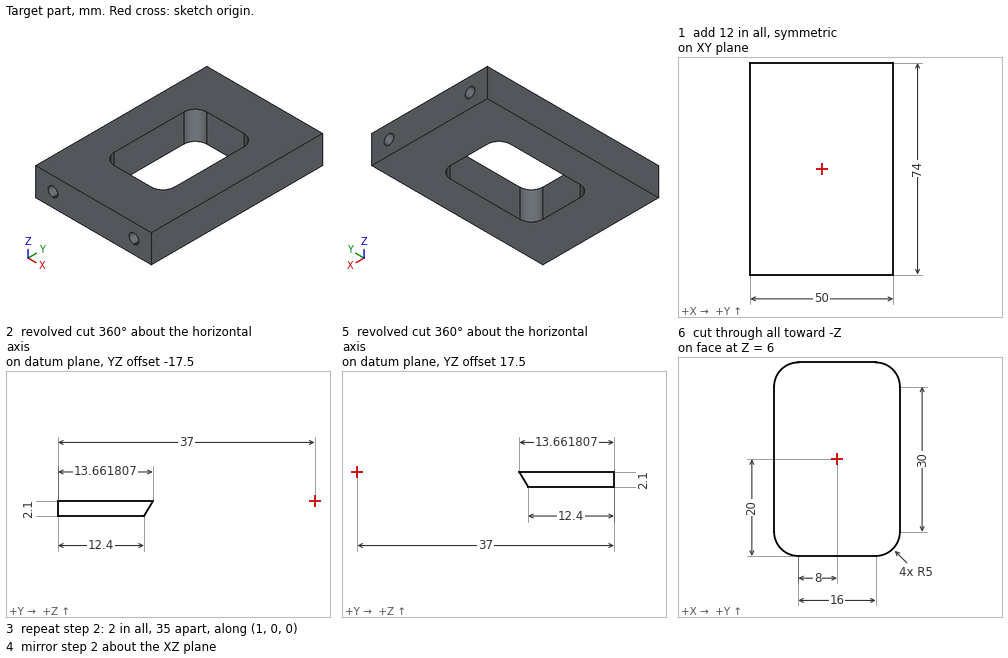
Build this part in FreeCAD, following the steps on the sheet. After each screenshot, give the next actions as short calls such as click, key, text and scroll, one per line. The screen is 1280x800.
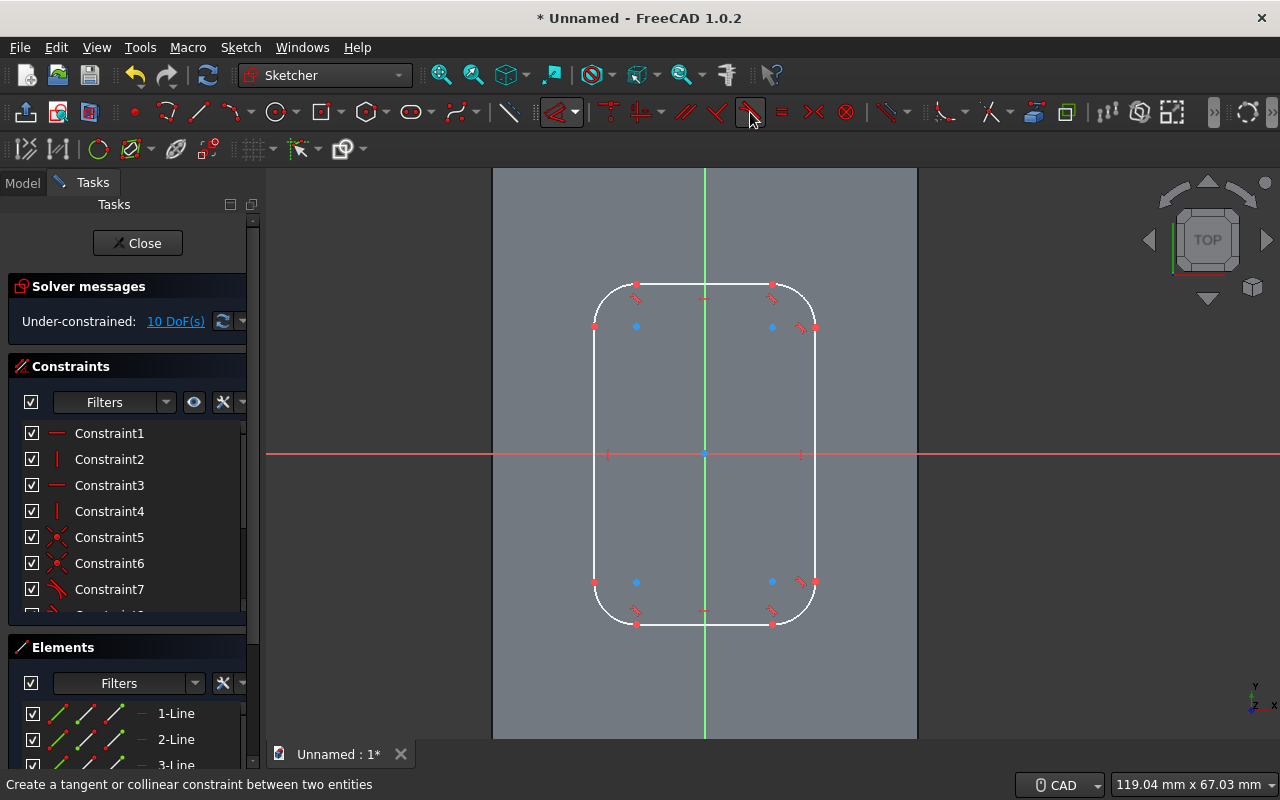
click(594, 403)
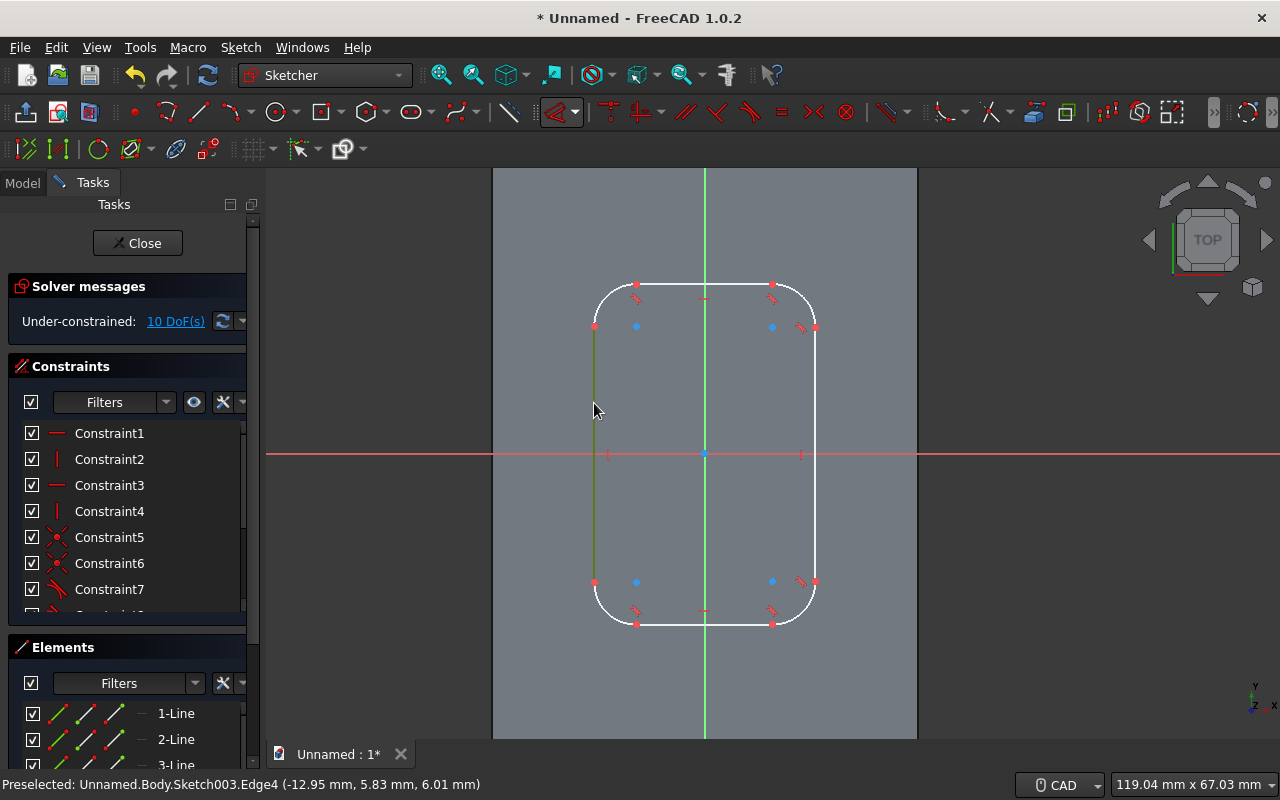
click(617, 289)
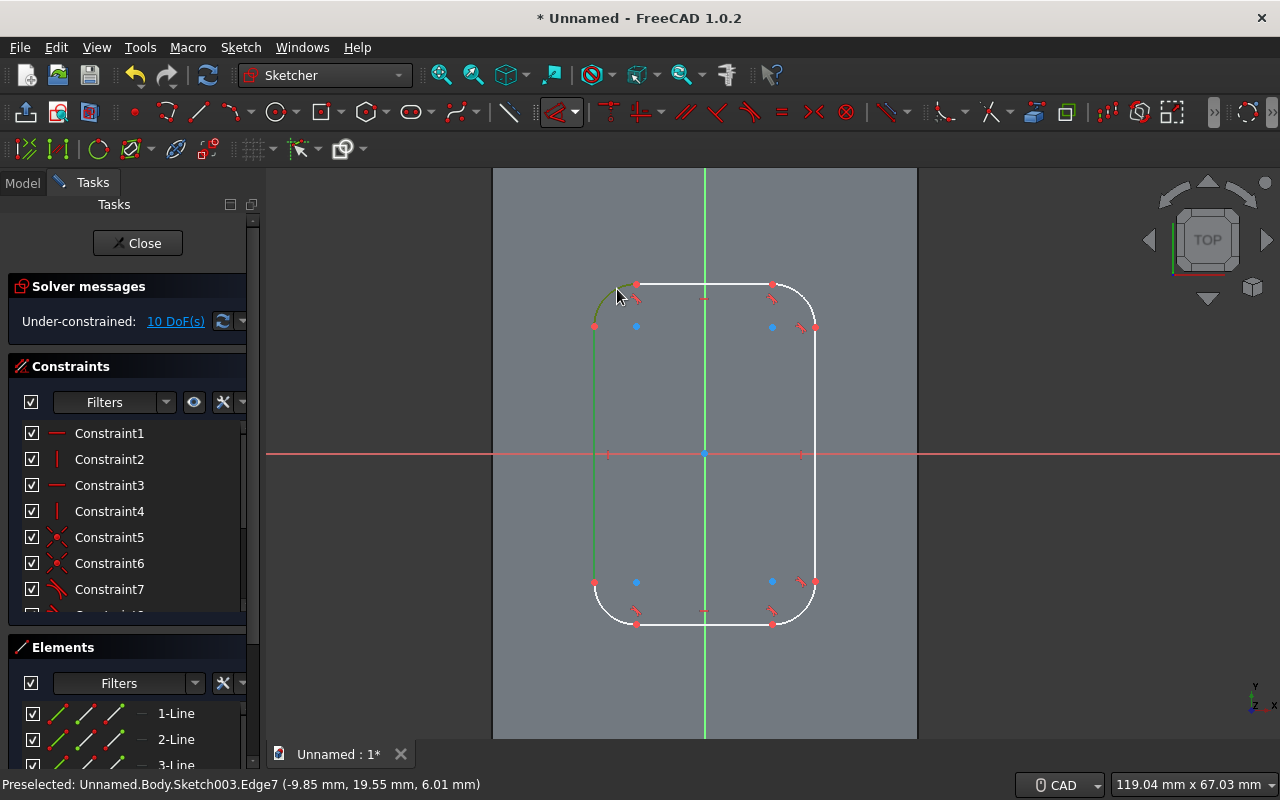
key(t)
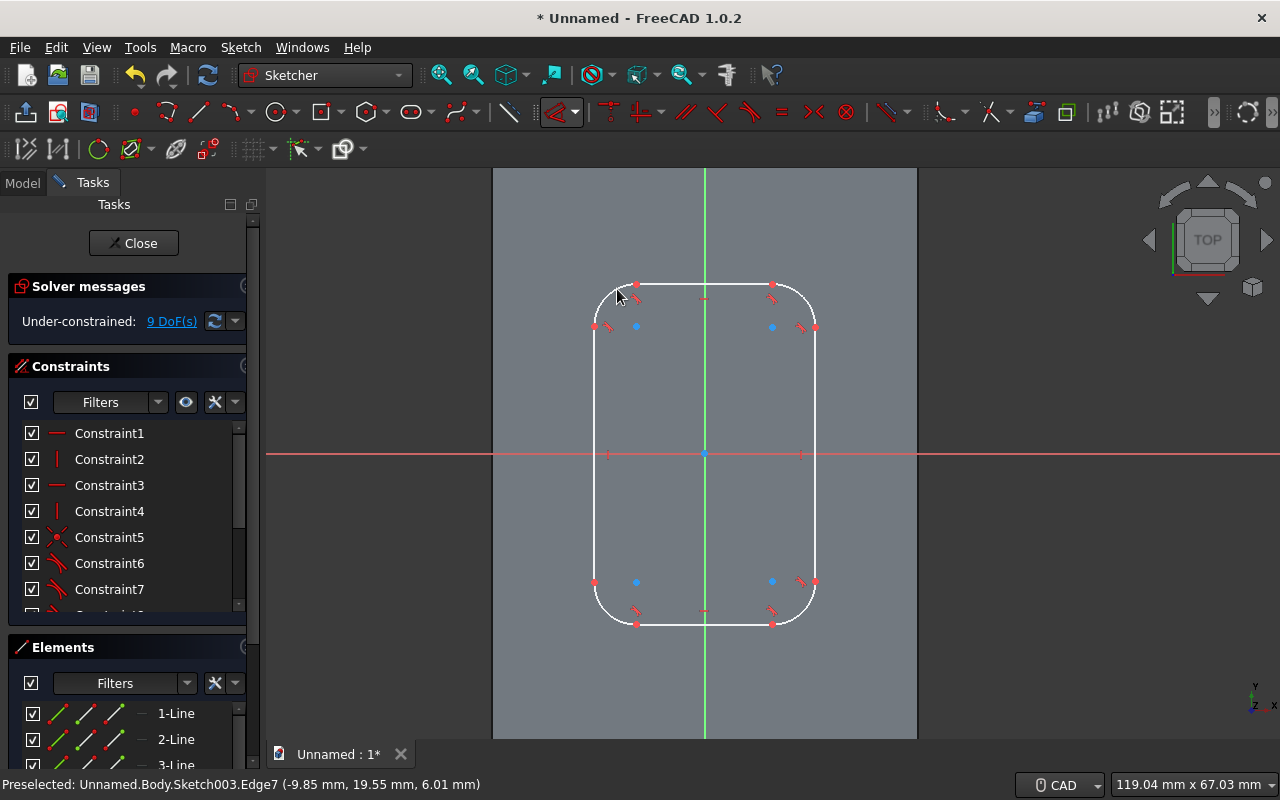
click(594, 403)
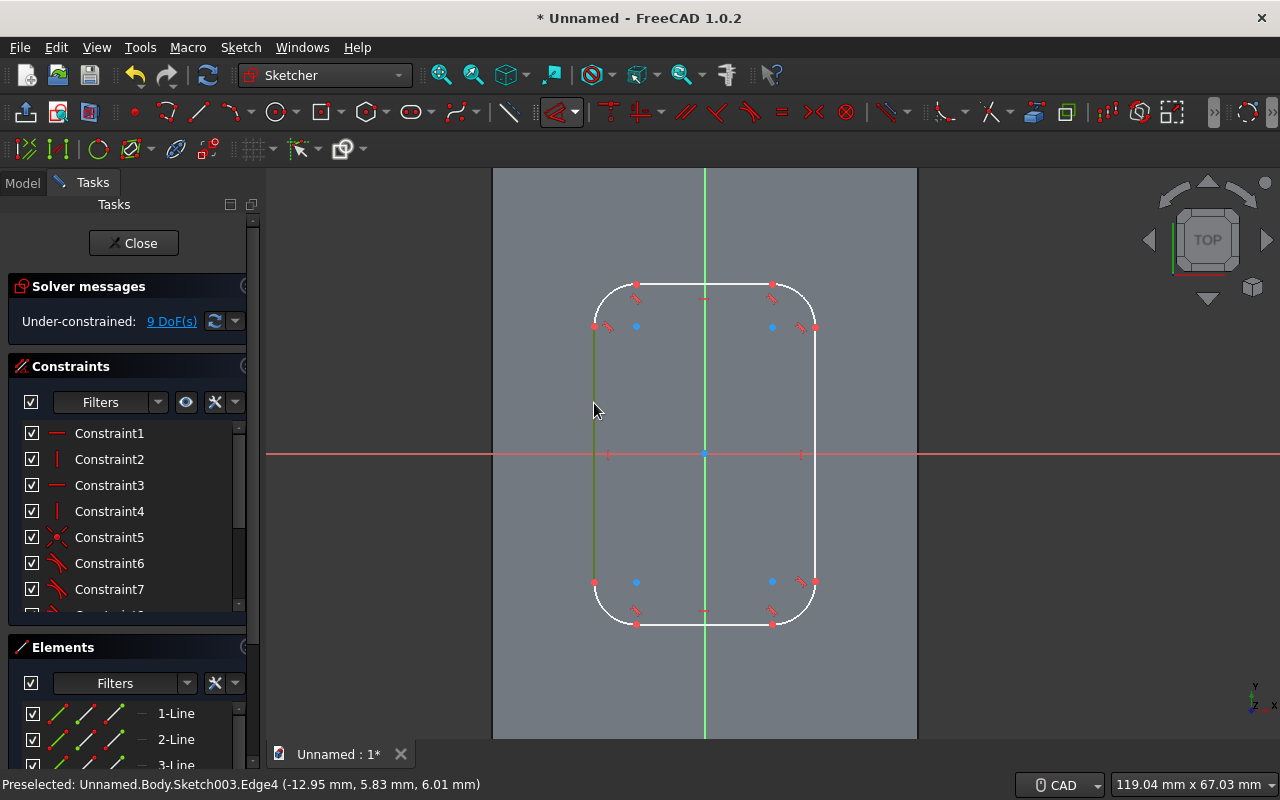
click(599, 602)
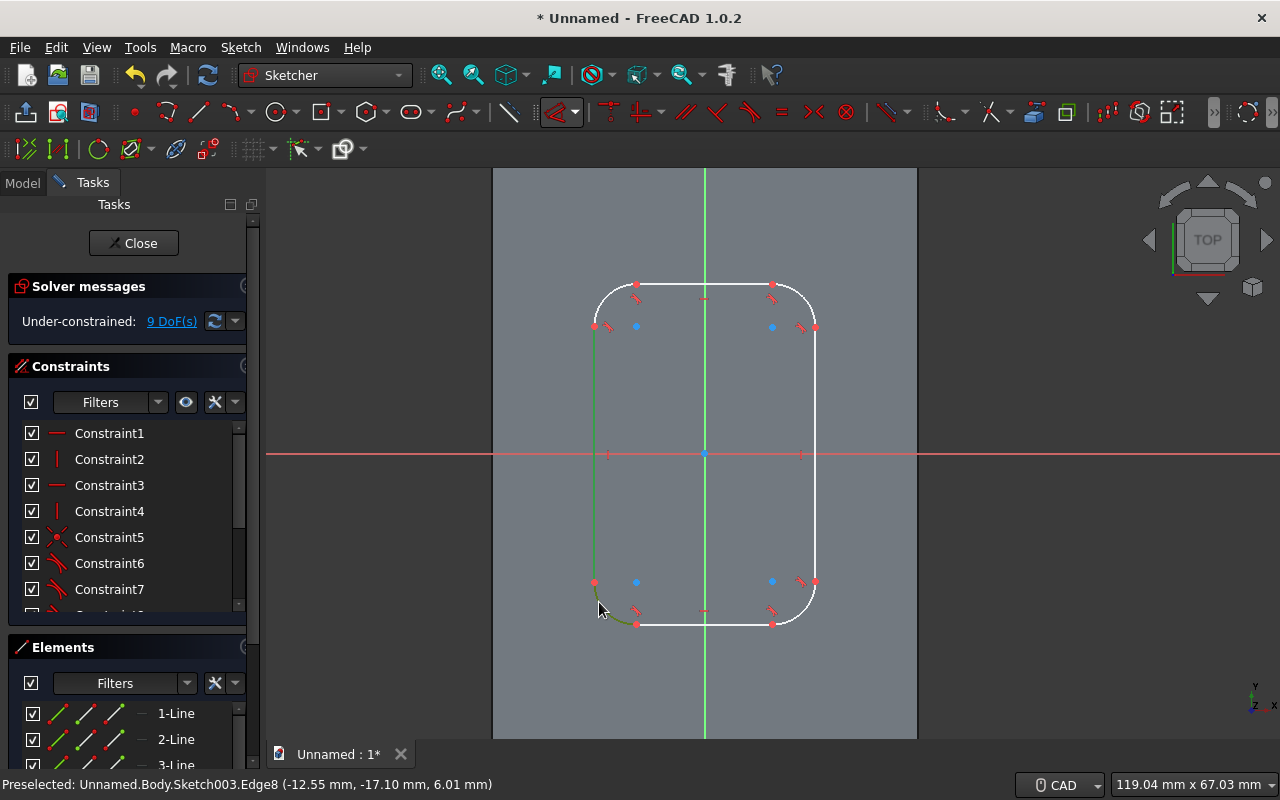
click(750, 112)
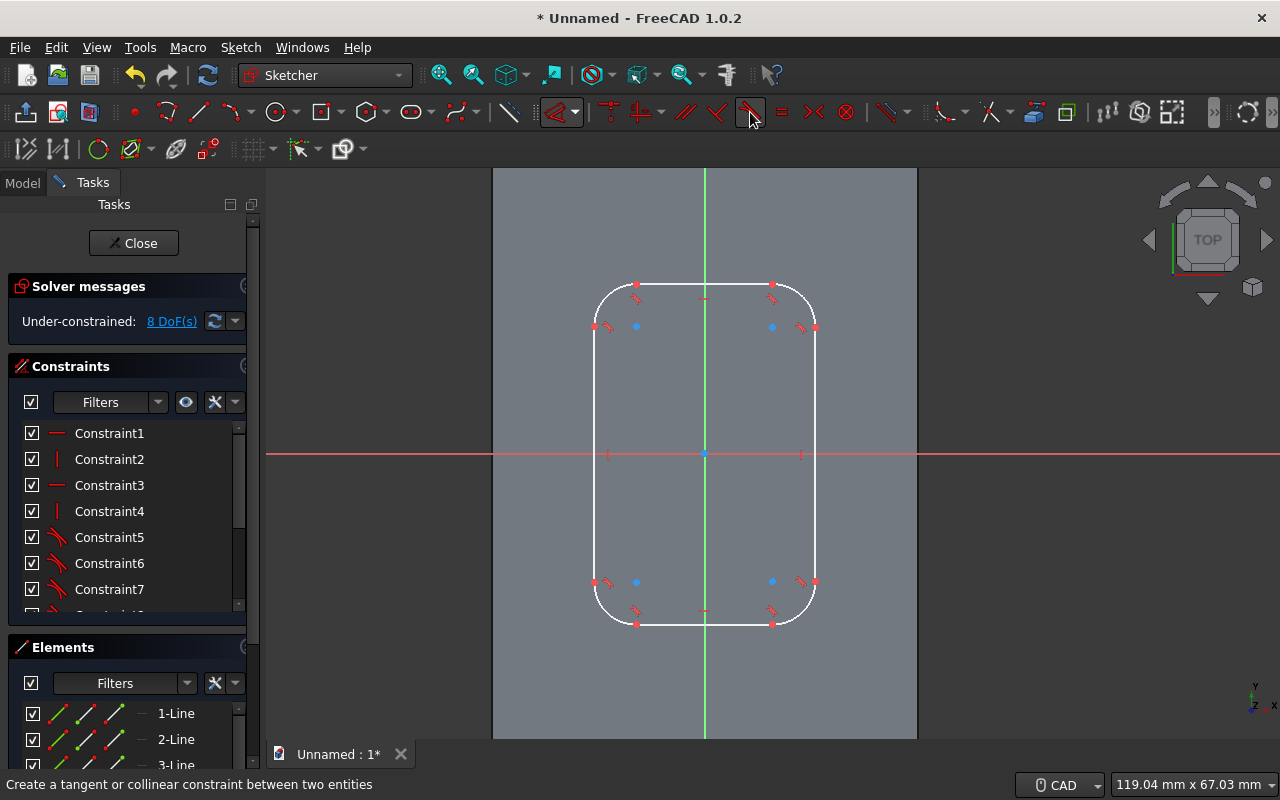
click(792, 620)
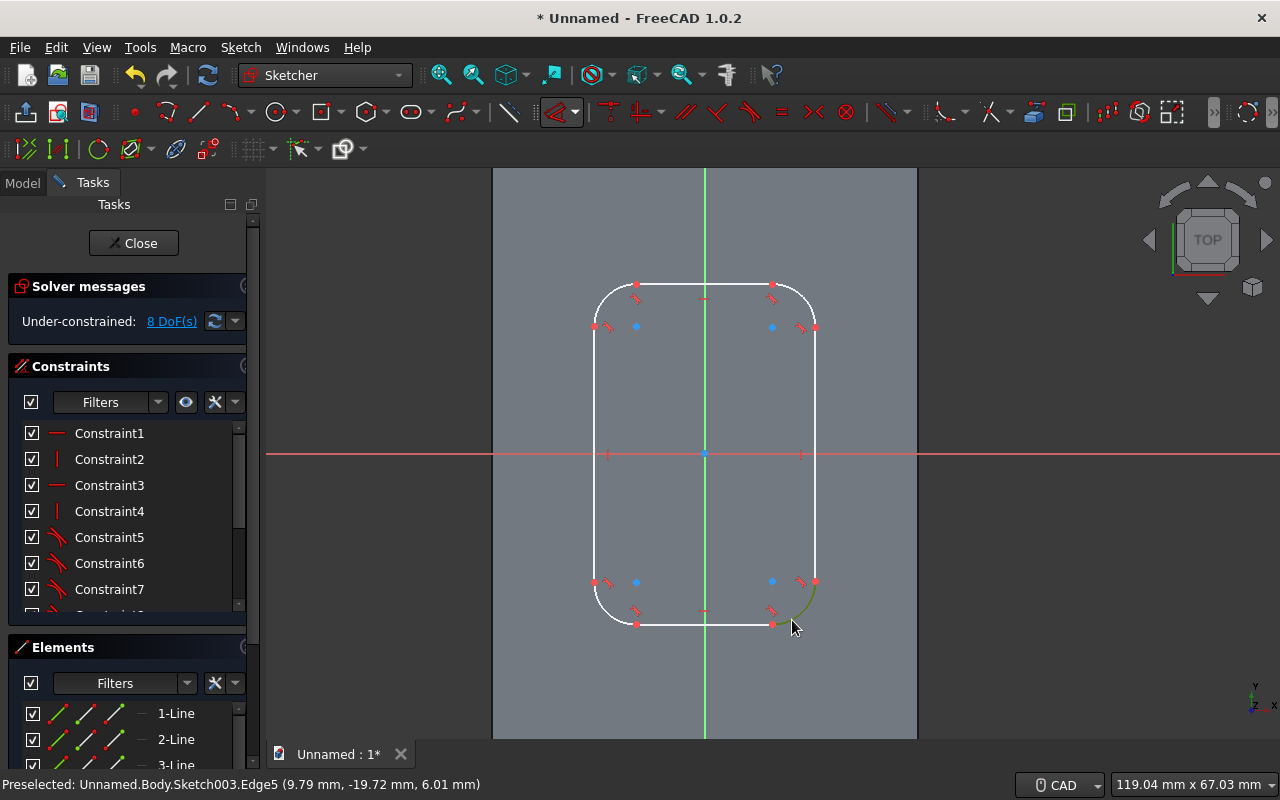
click(811, 308)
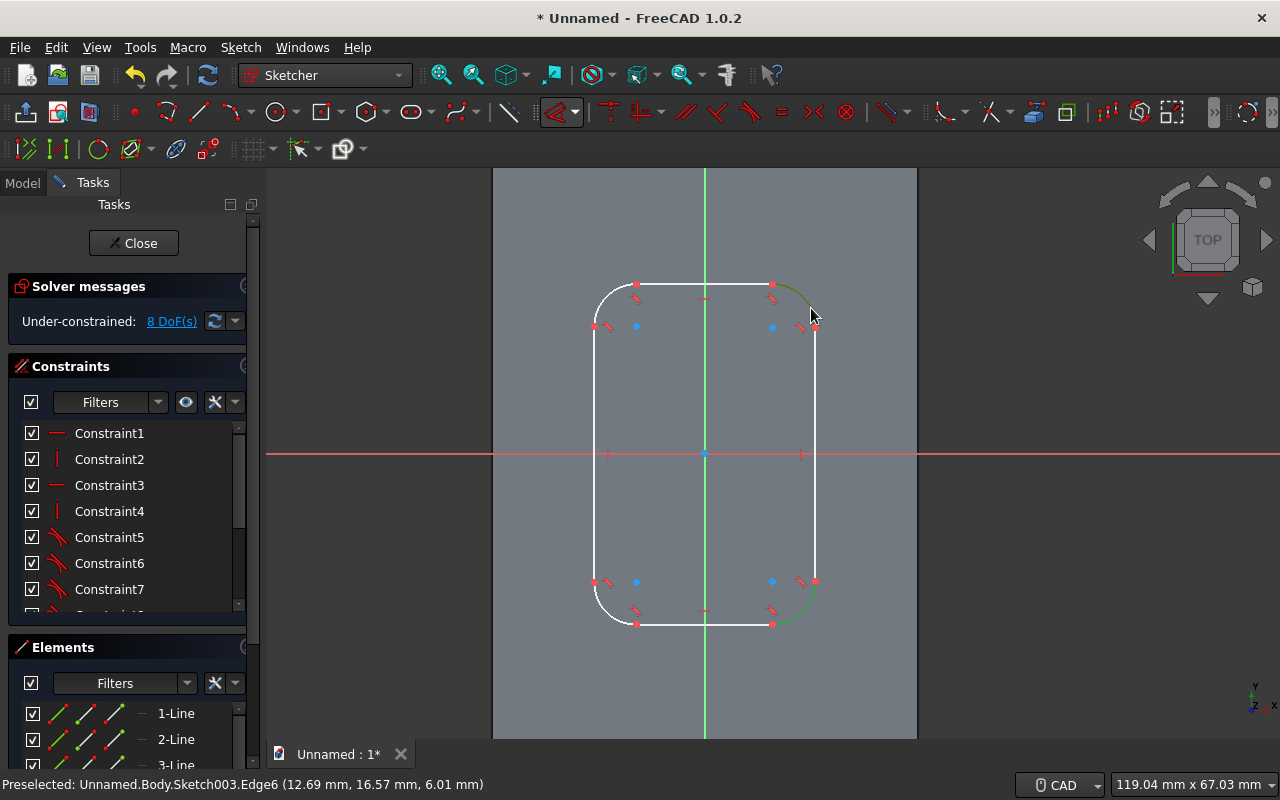
click(618, 289)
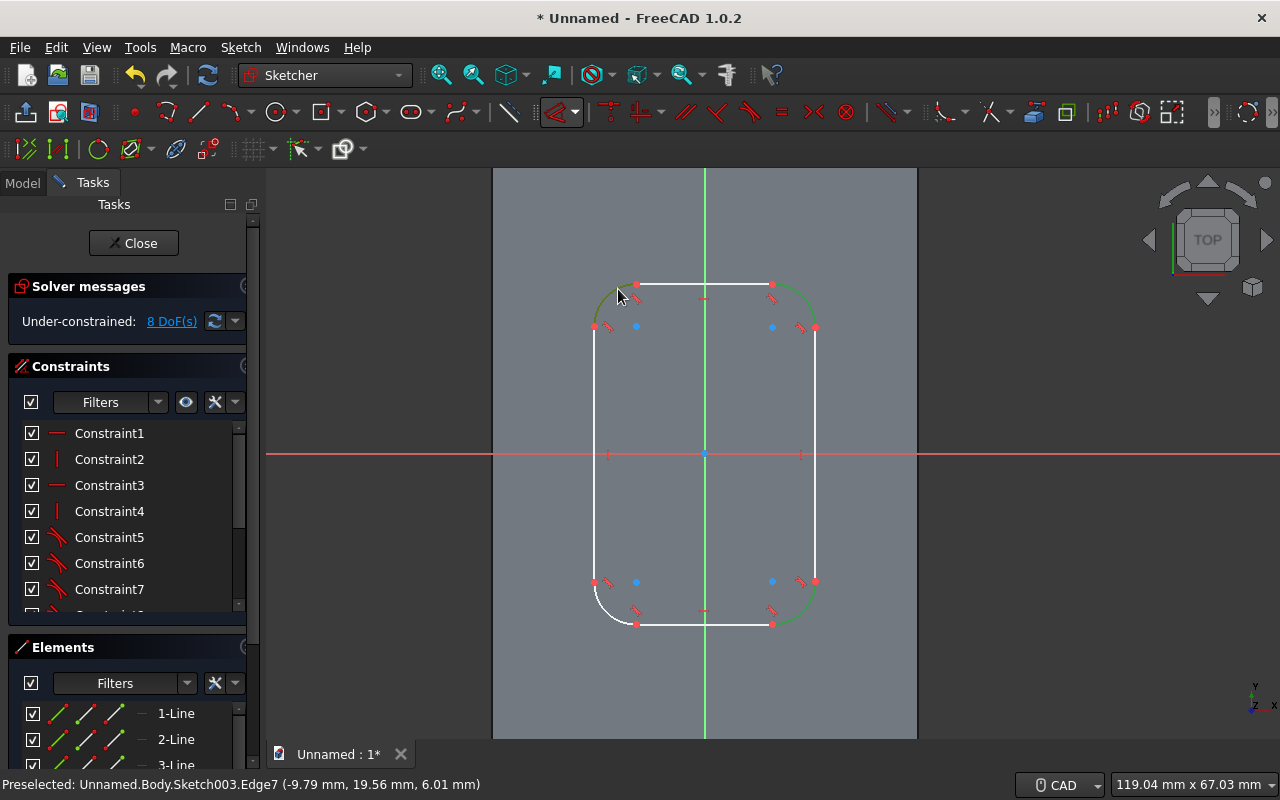
click(599, 602)